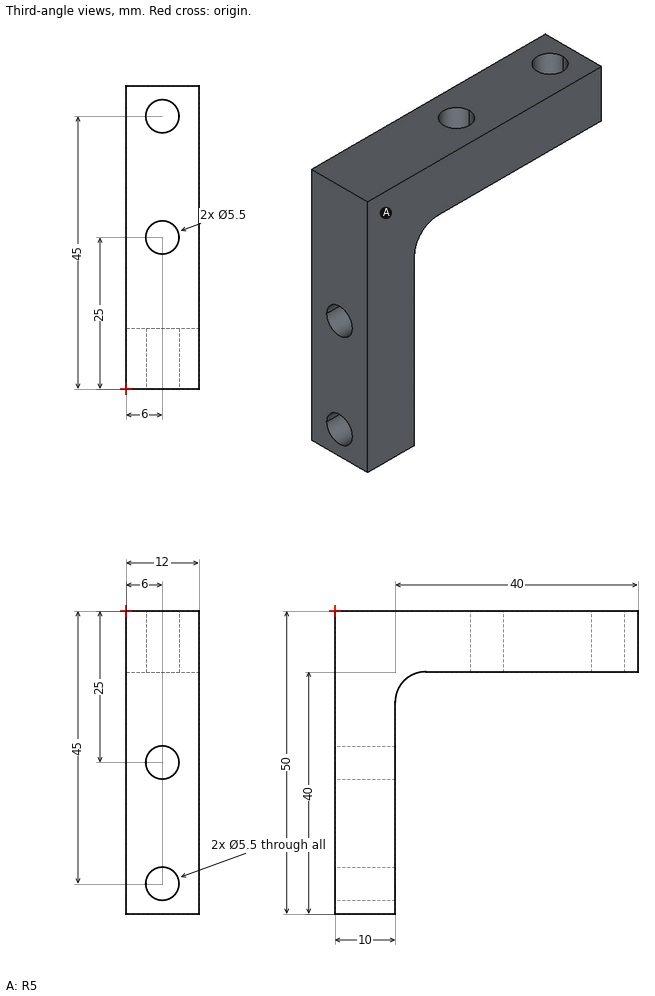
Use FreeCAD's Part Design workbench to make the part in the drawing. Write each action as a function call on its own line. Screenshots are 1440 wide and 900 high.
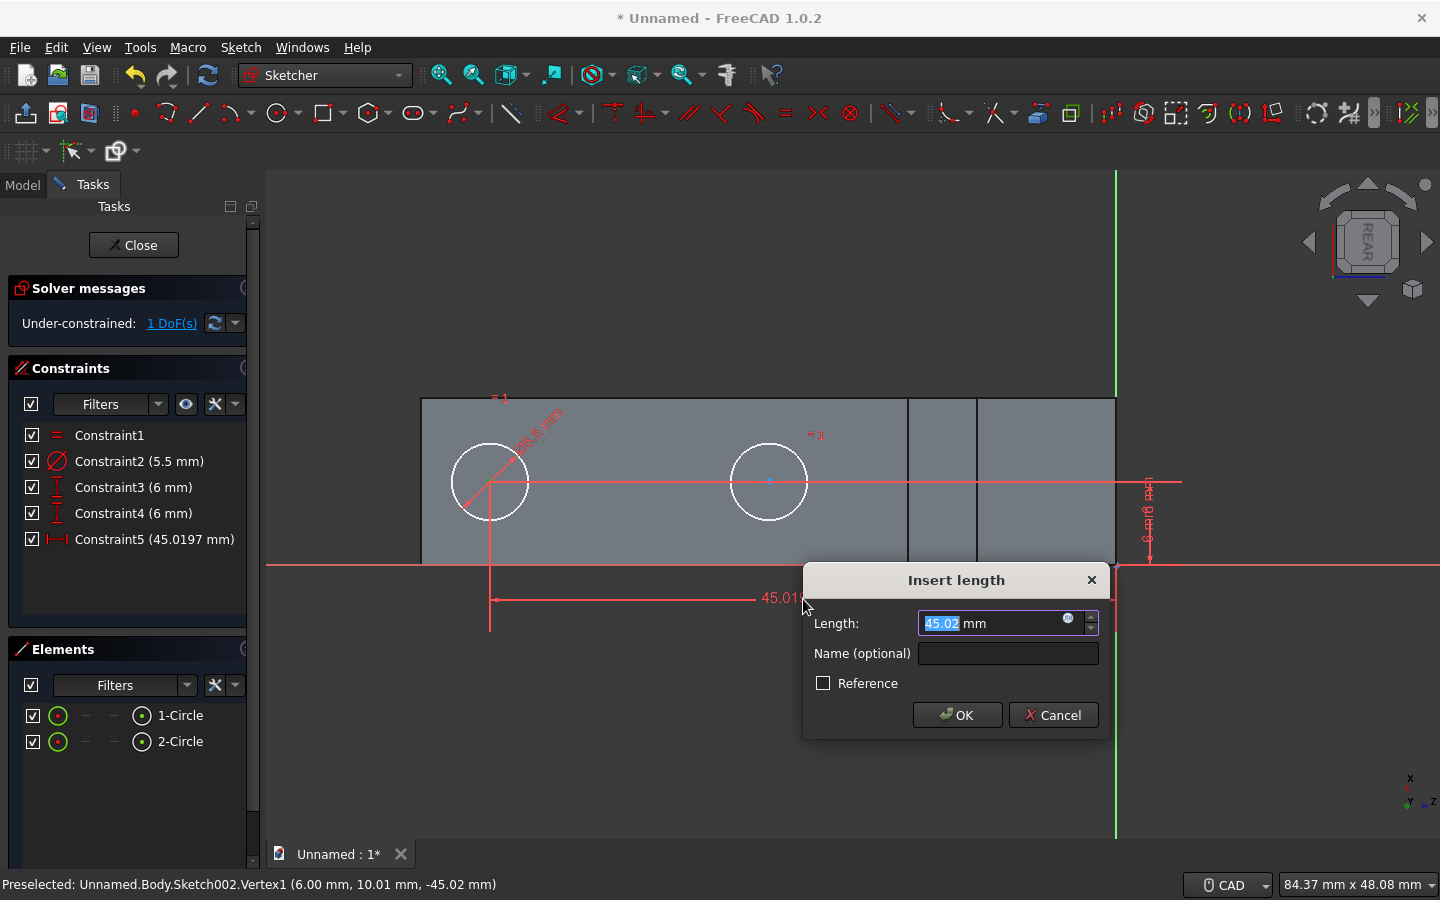
text(45)
key(Return)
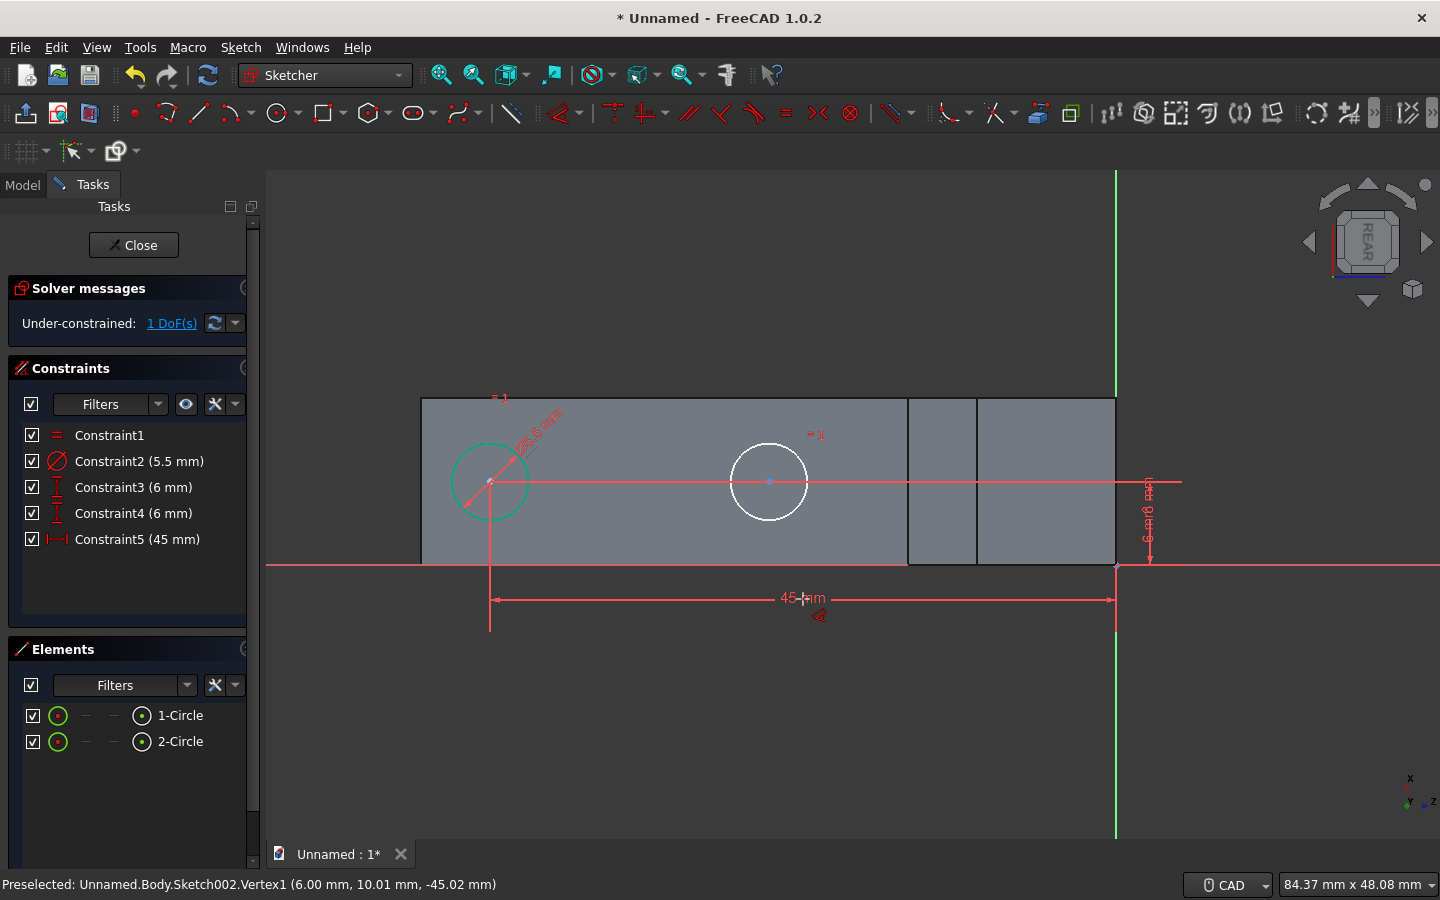
click(769, 482)
click(943, 599)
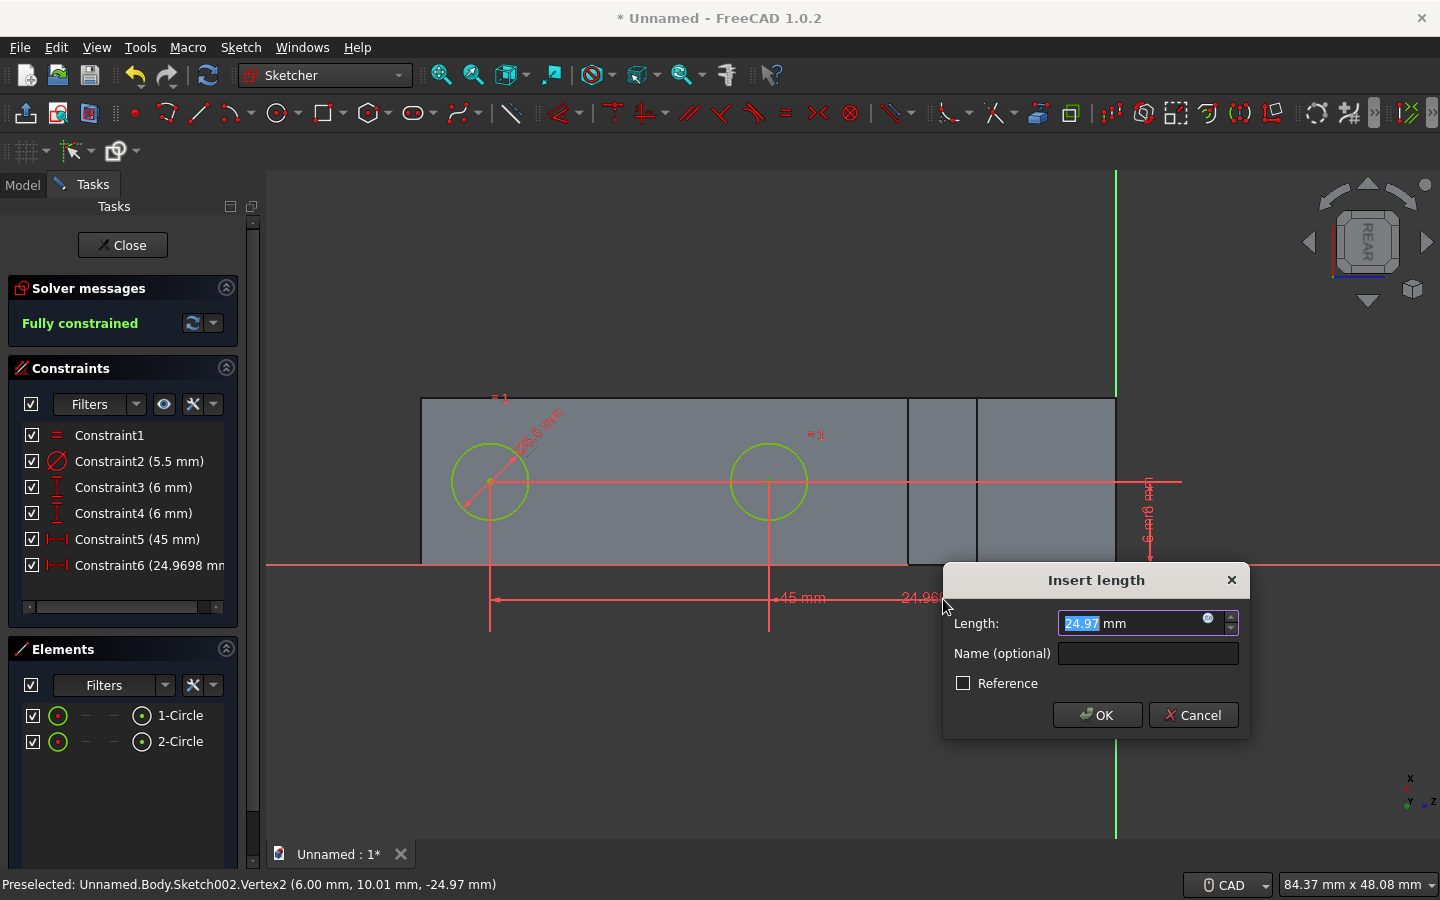
text(25)
key(Return)
key(Escape)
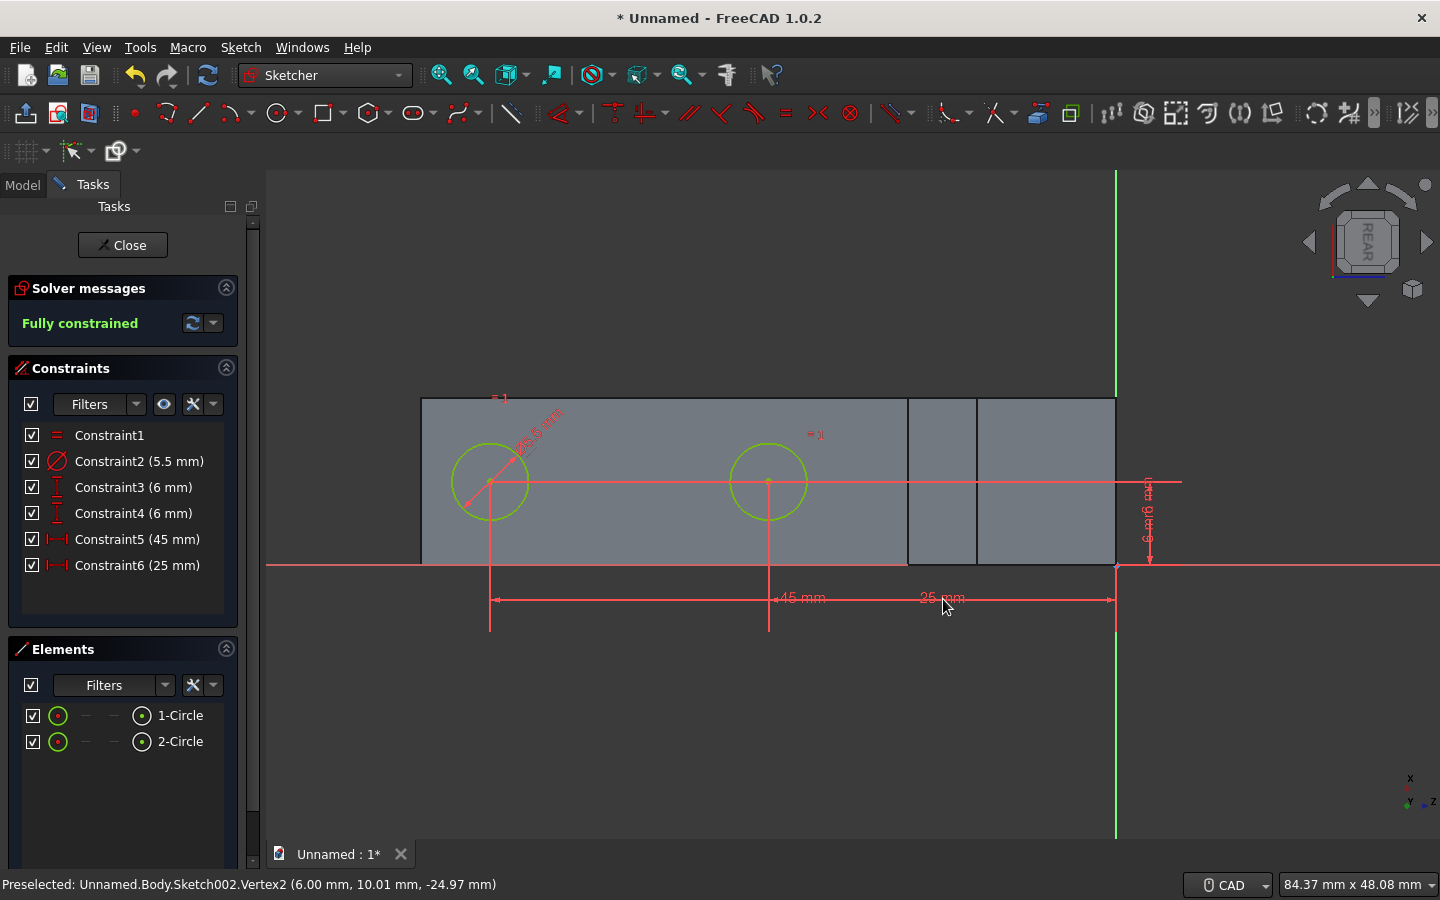
click(123, 245)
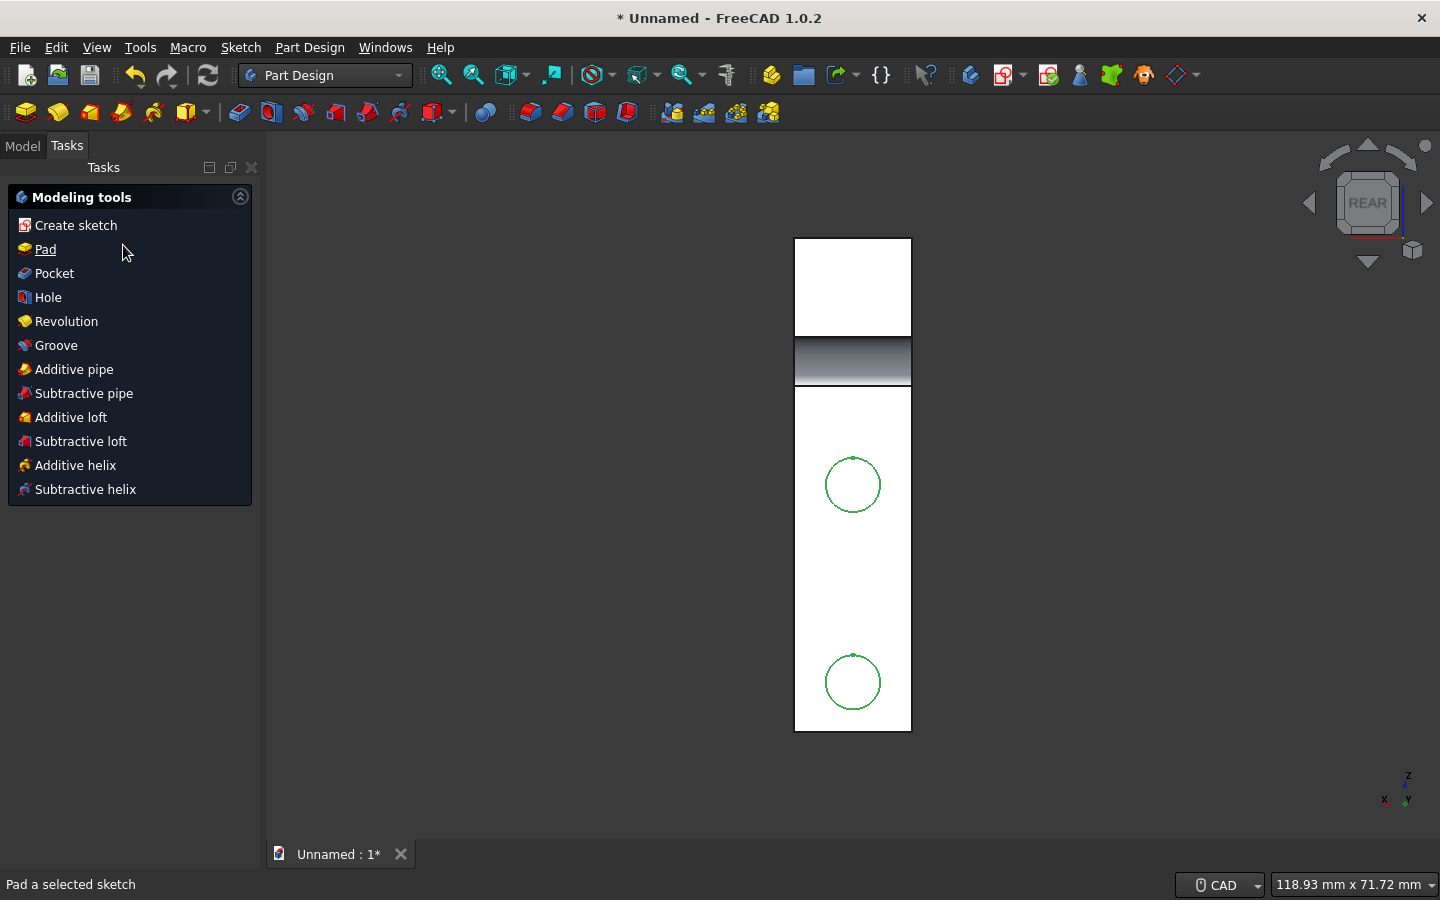
click(272, 112)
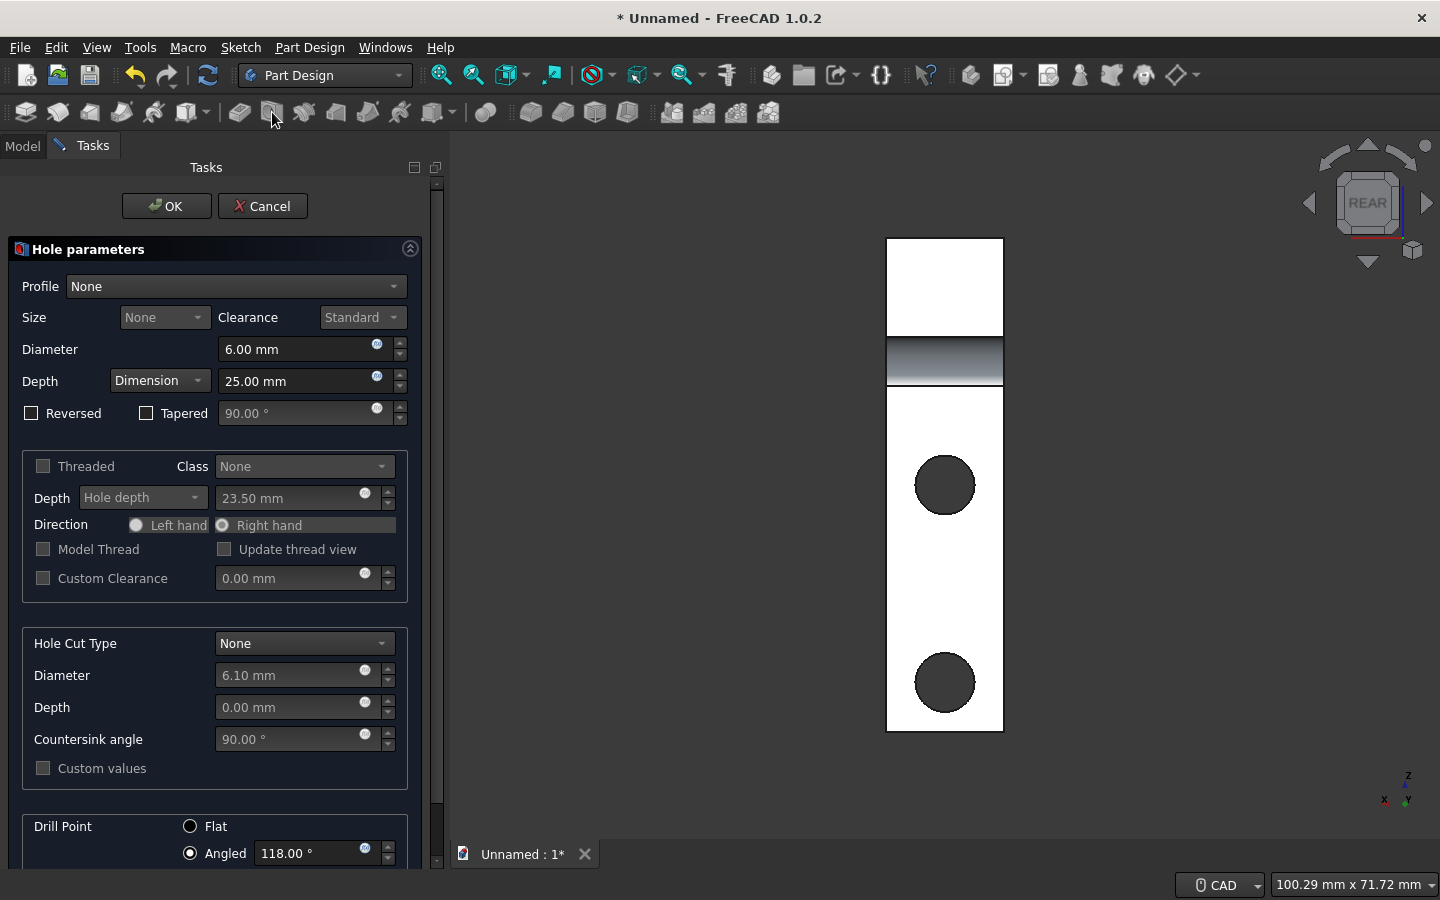
triple_click(305, 349)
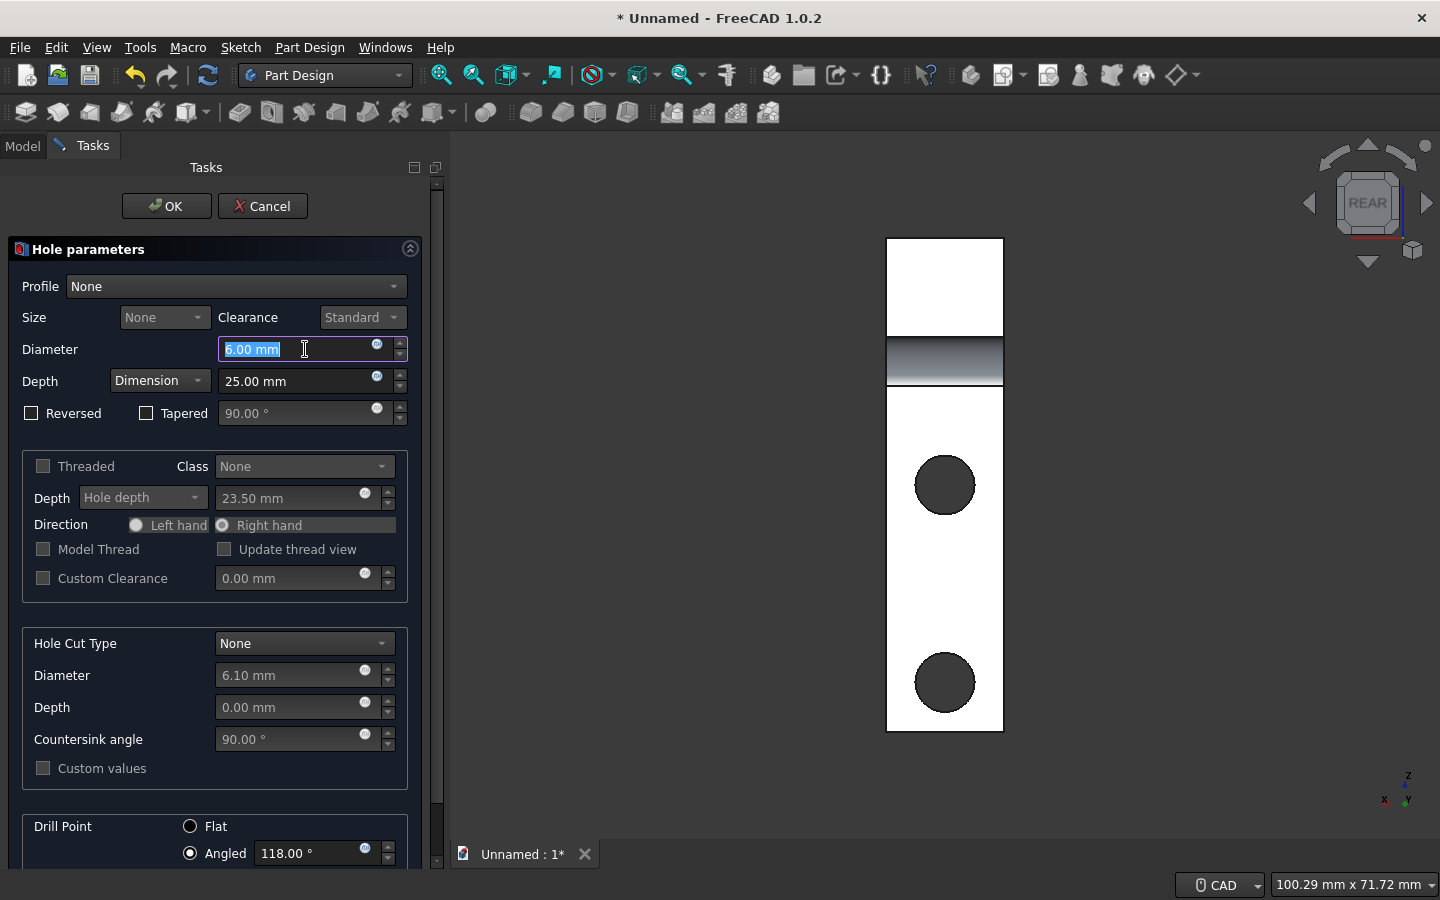
text(5.5)
key(Tab)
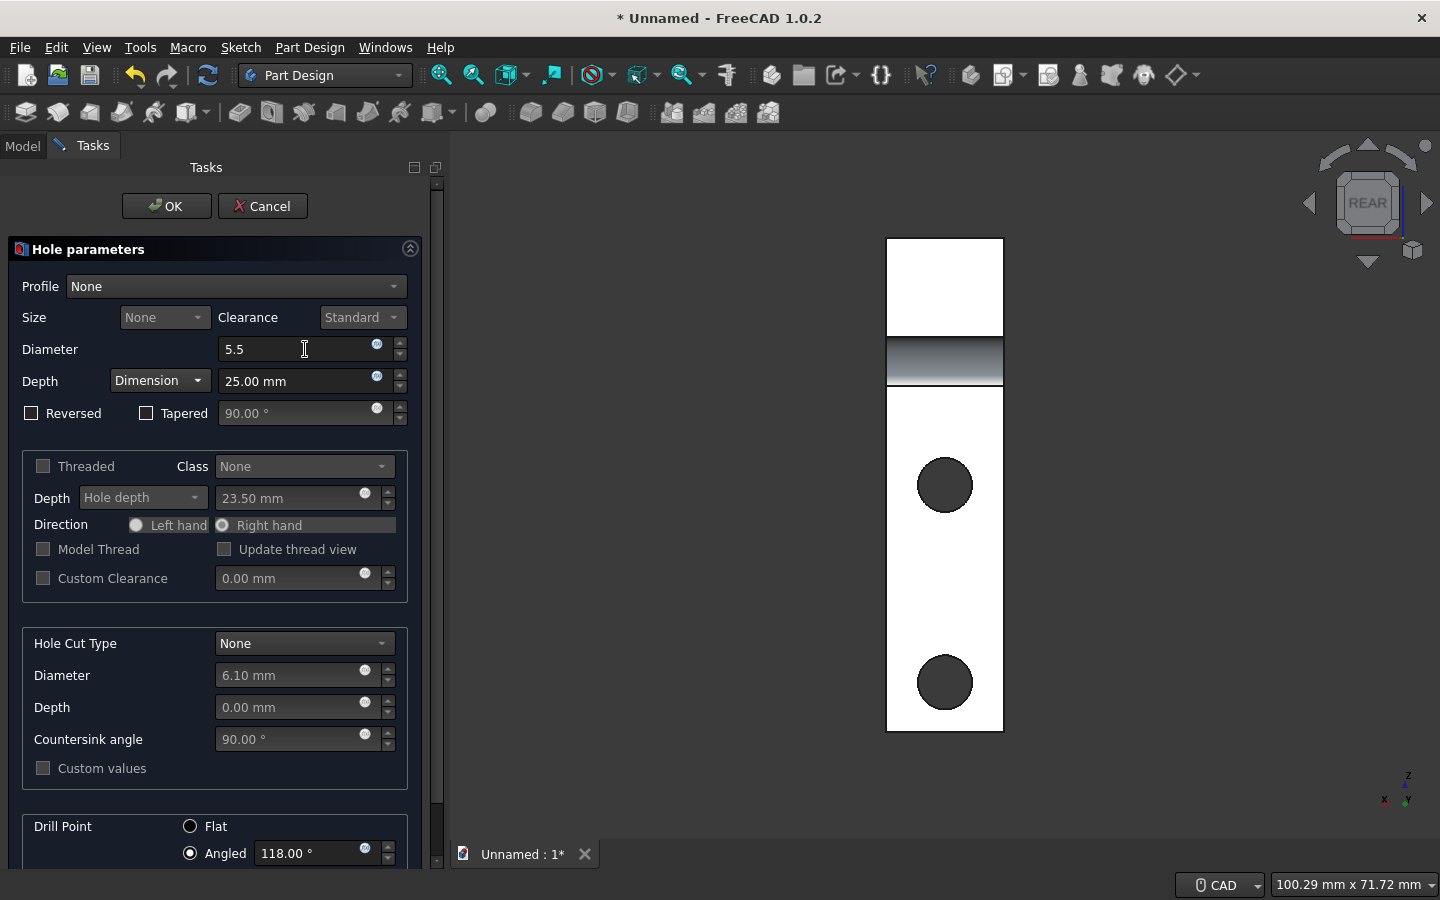
click(161, 380)